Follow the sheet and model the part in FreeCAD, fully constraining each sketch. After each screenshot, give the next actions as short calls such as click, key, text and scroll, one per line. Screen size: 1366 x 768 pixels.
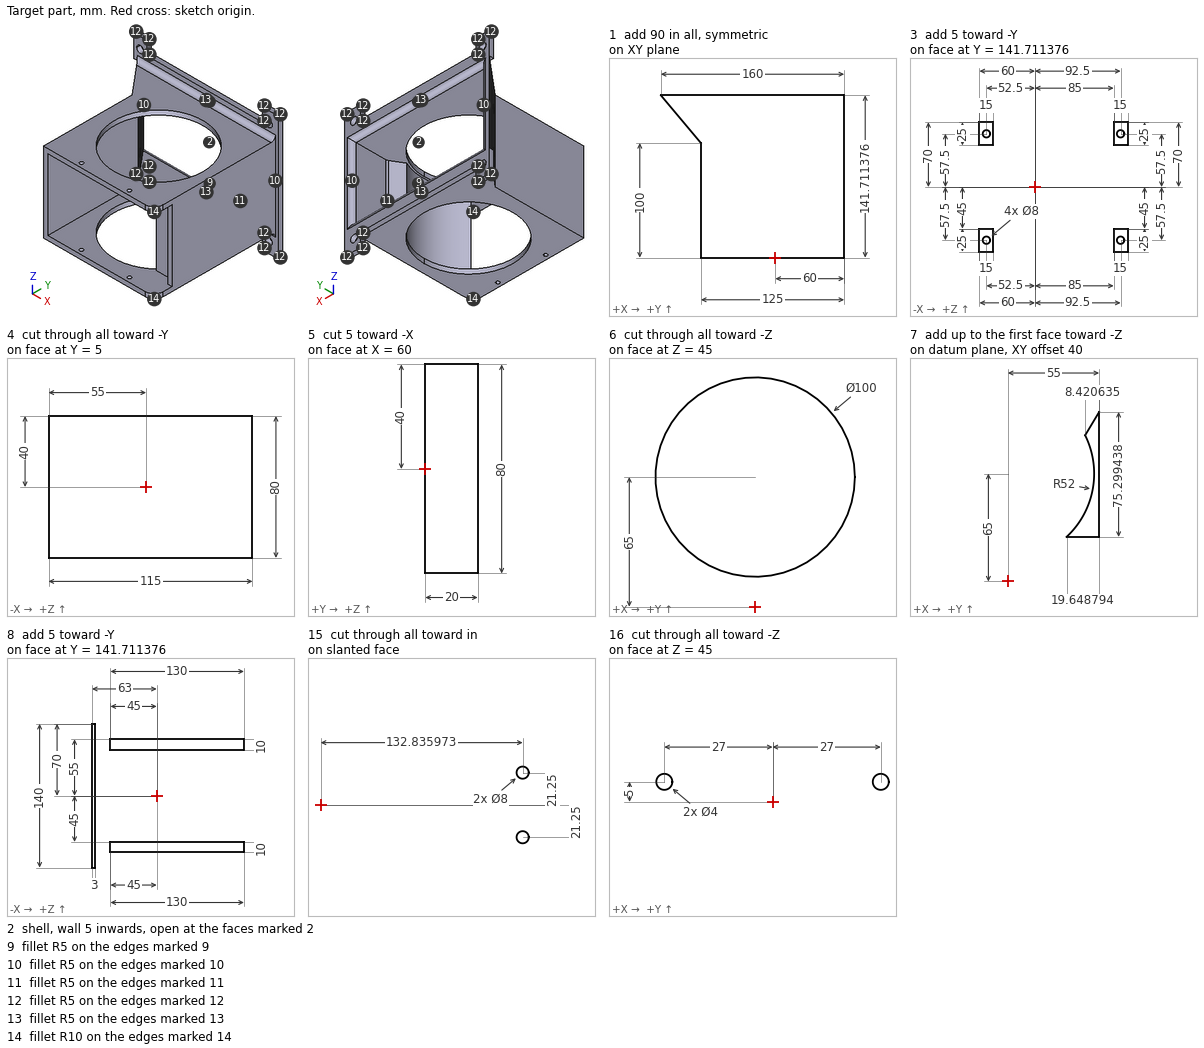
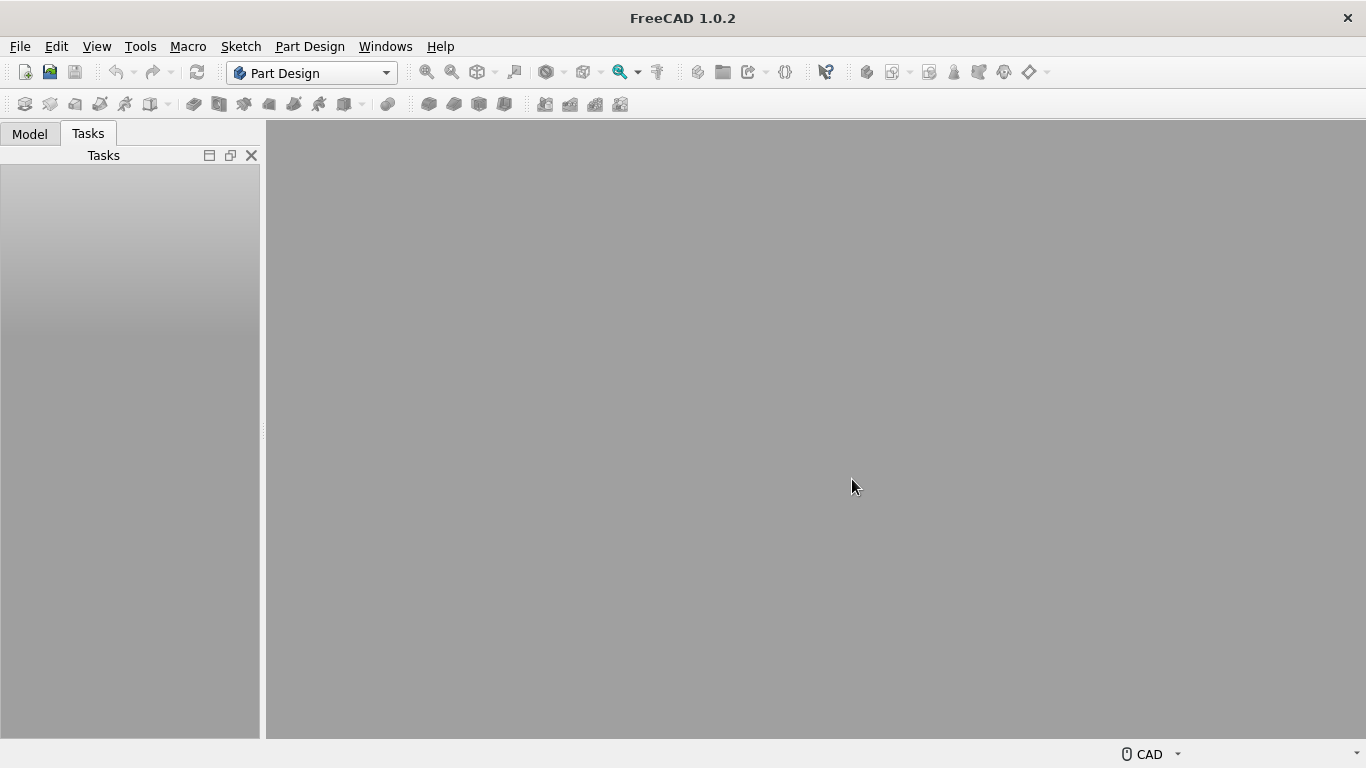
key(ctrl+n)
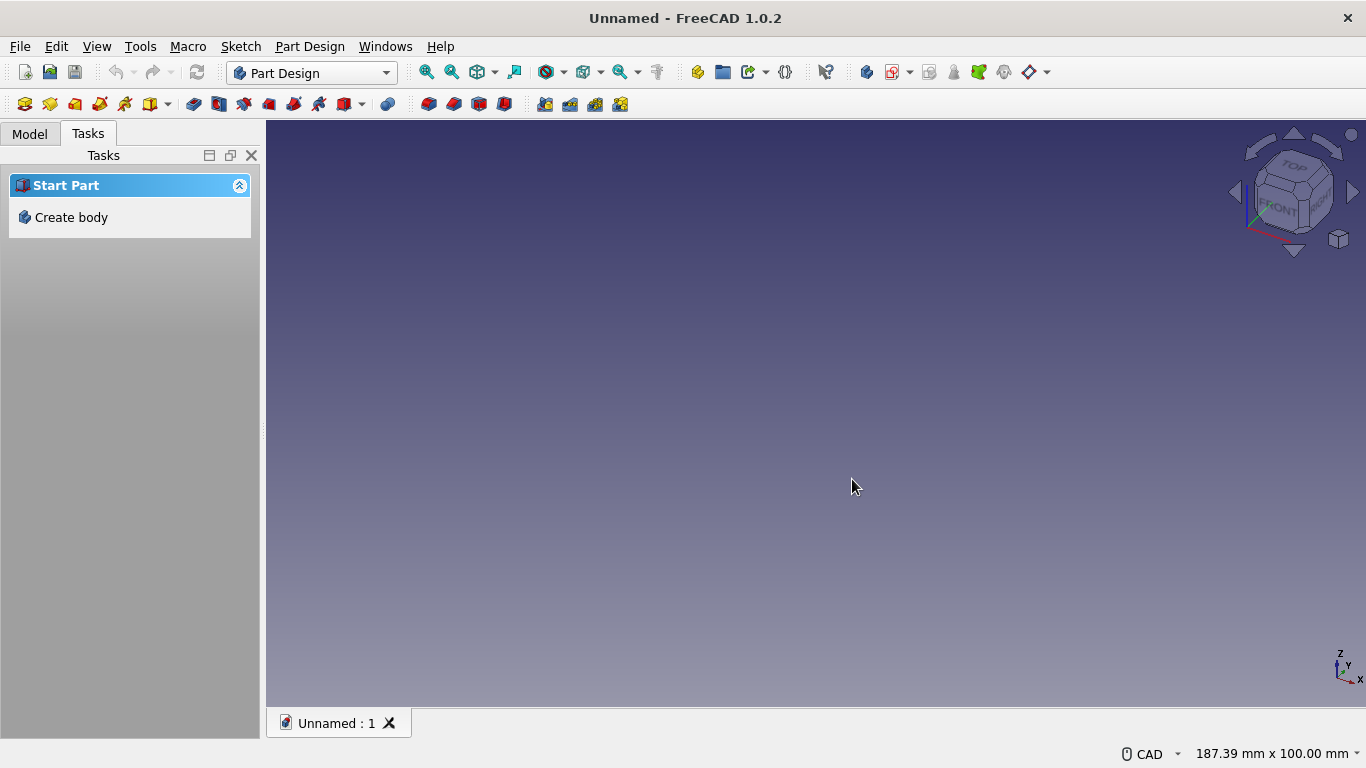
click(892, 72)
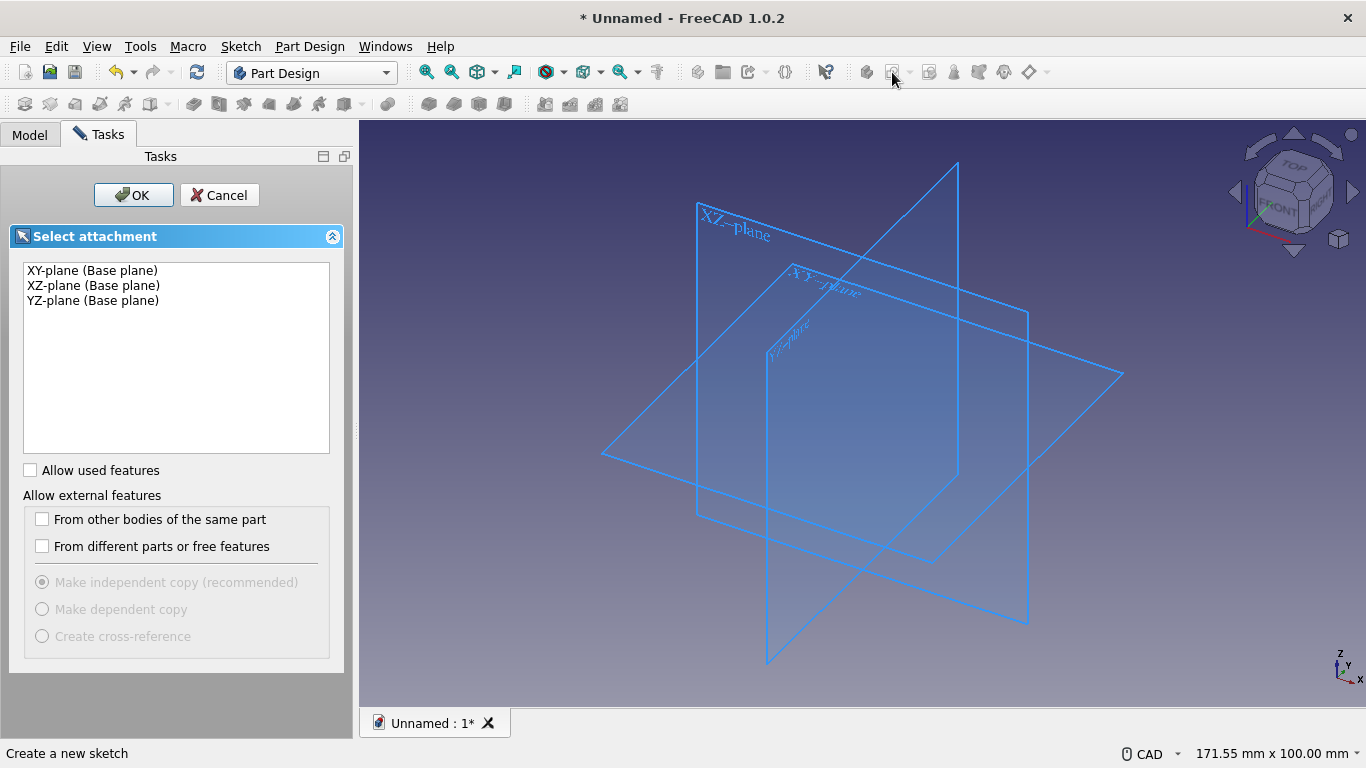
click(84, 270)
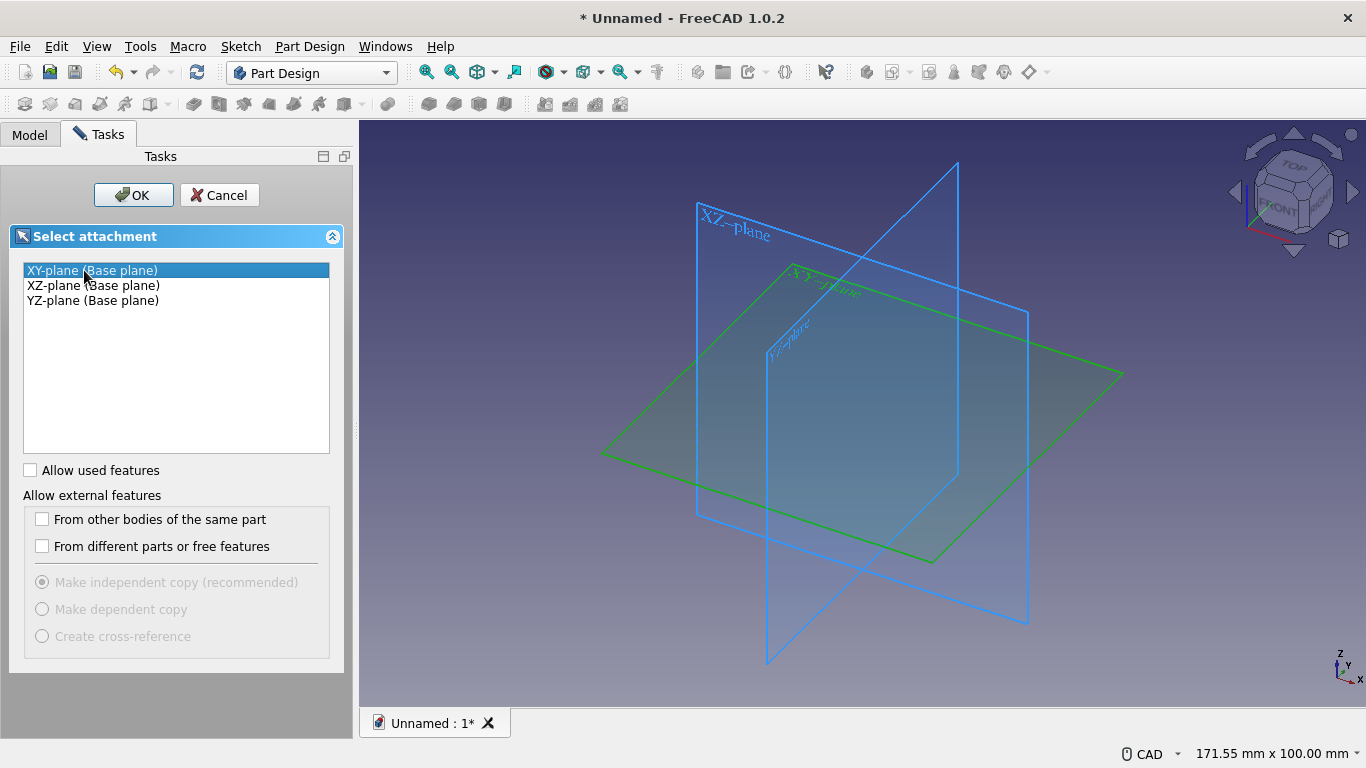
click(134, 195)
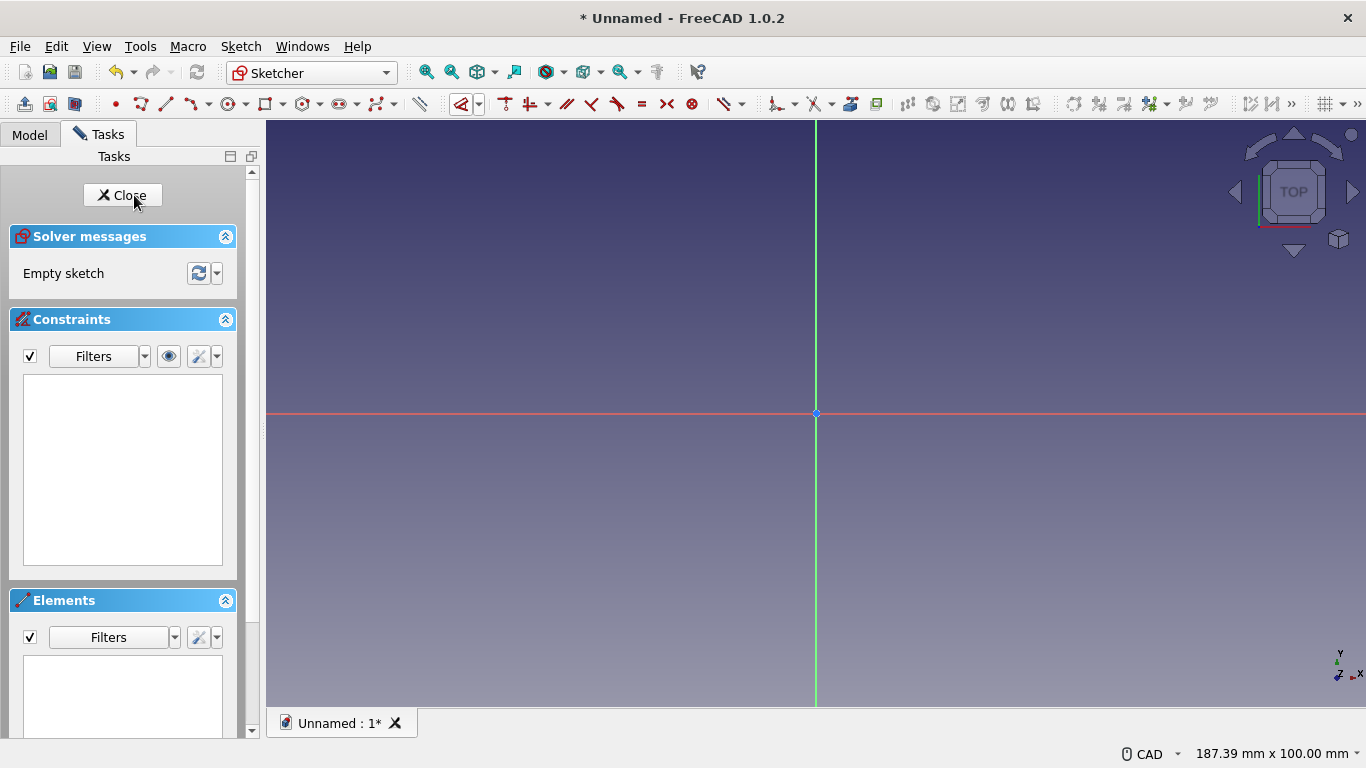
scroll(787, 679, down, 4)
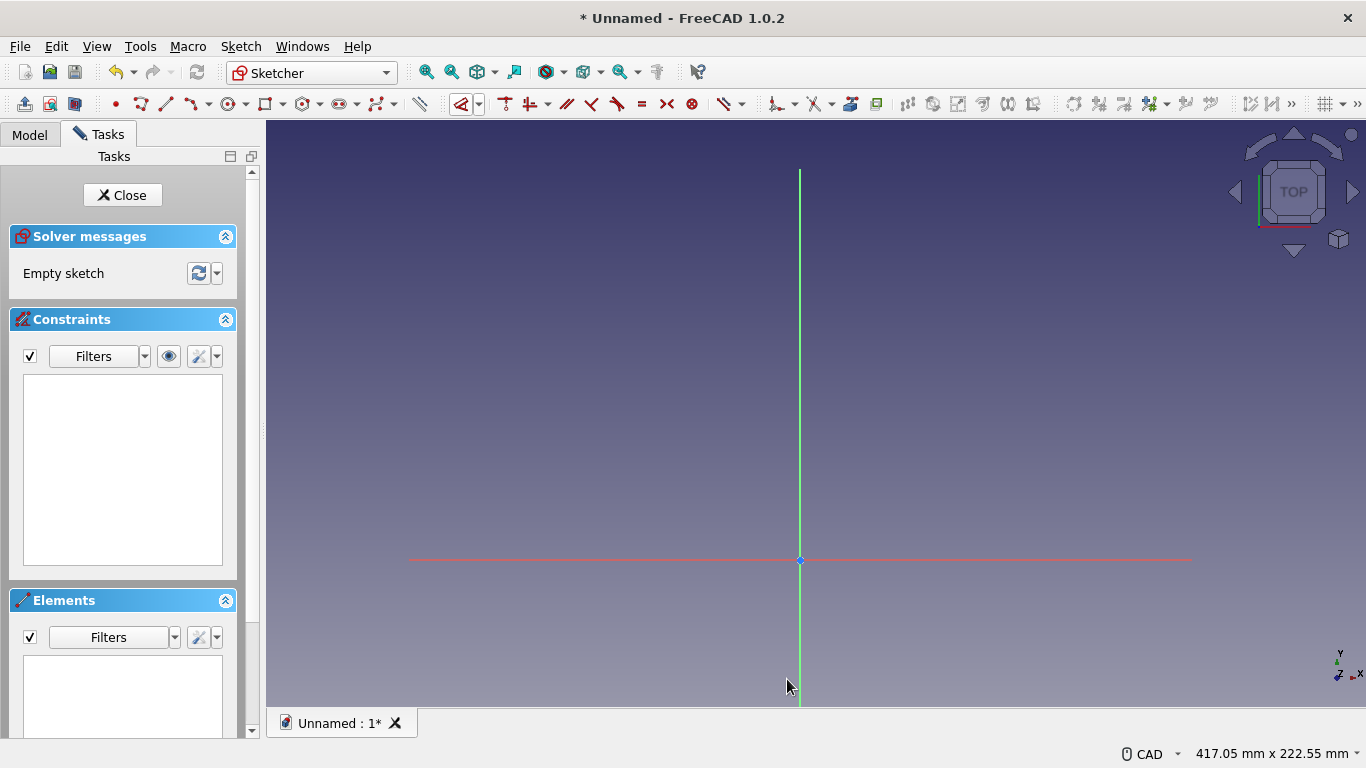
key(g)
key(m)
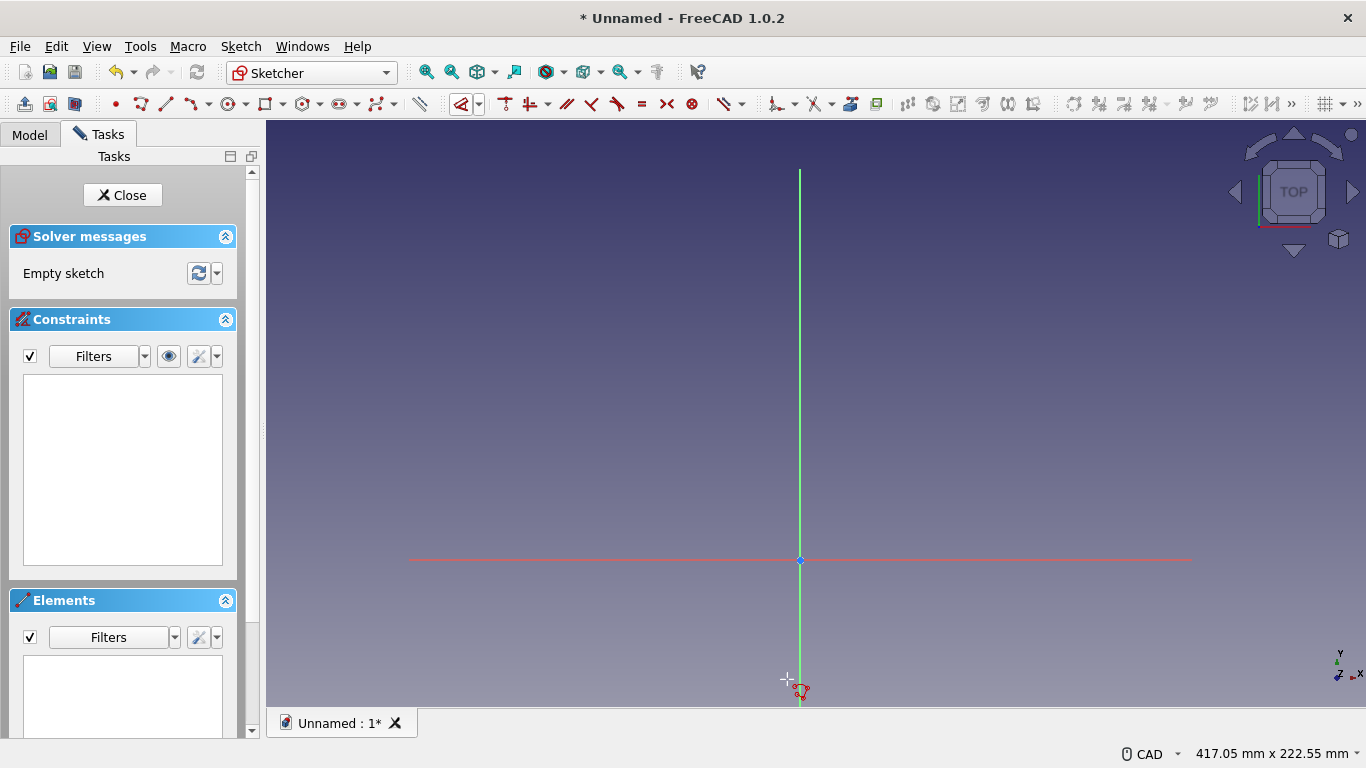
click(959, 560)
click(959, 186)
click(537, 186)
click(629, 296)
click(629, 551)
click(959, 560)
key(Escape)
key(Escape)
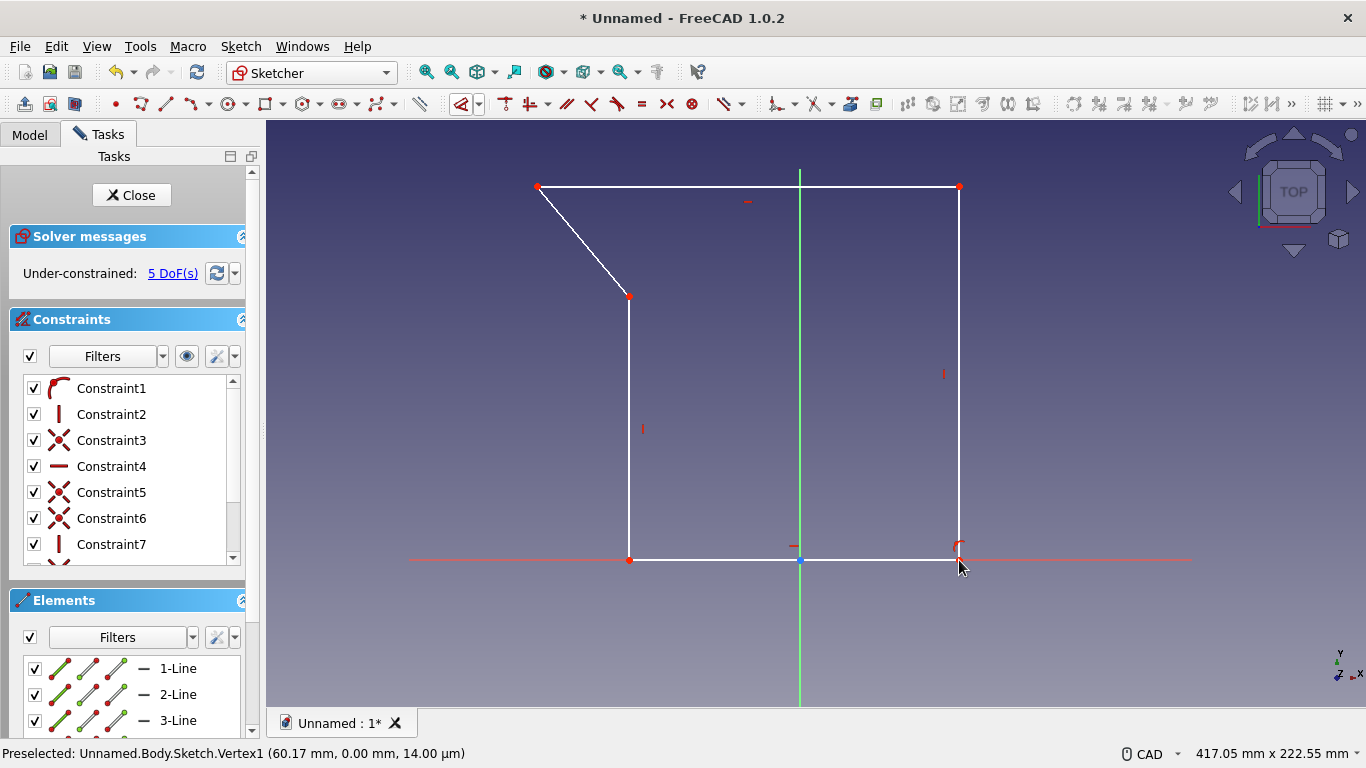
click(832, 187)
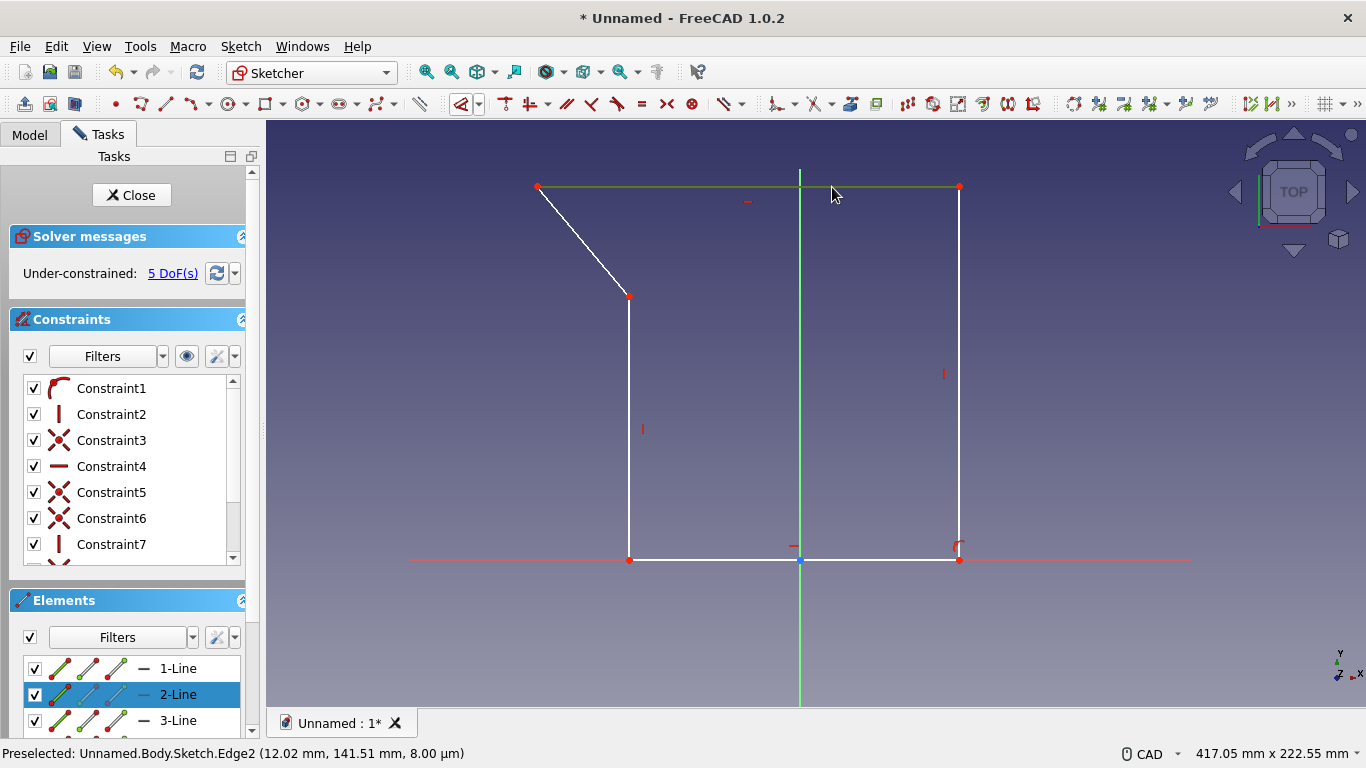
click(478, 104)